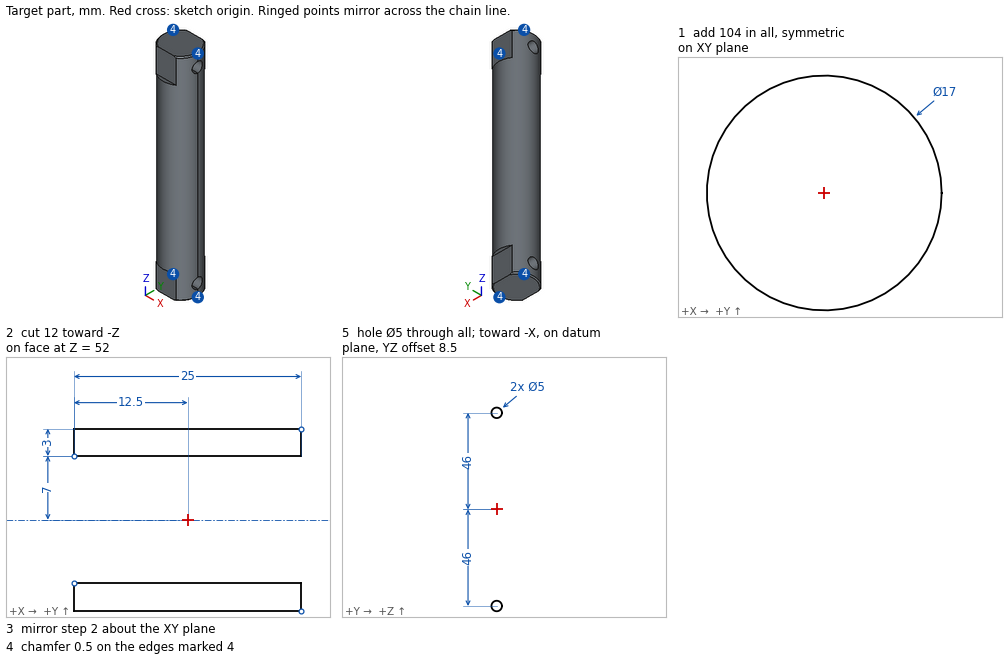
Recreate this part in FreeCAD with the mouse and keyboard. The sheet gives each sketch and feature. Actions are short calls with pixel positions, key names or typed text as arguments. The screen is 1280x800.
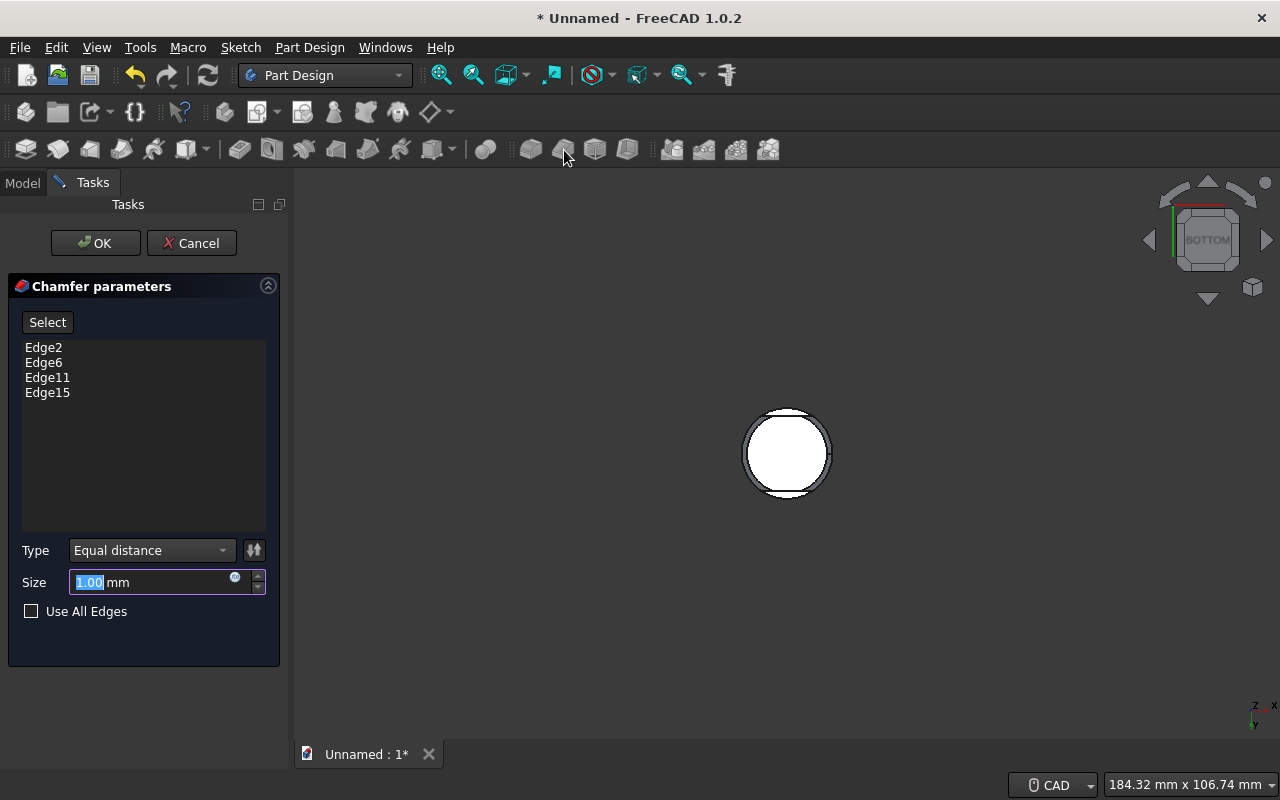
text(0.5)
key(Tab)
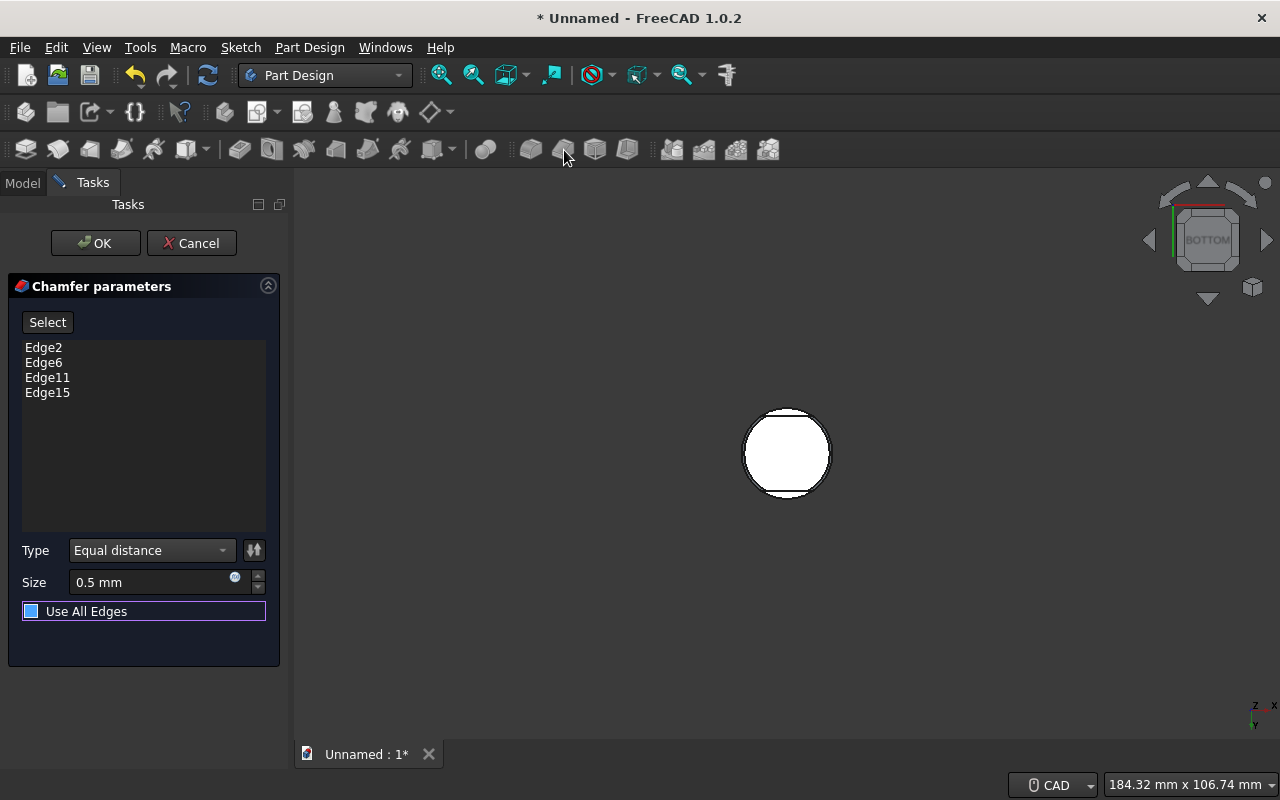
click(96, 243)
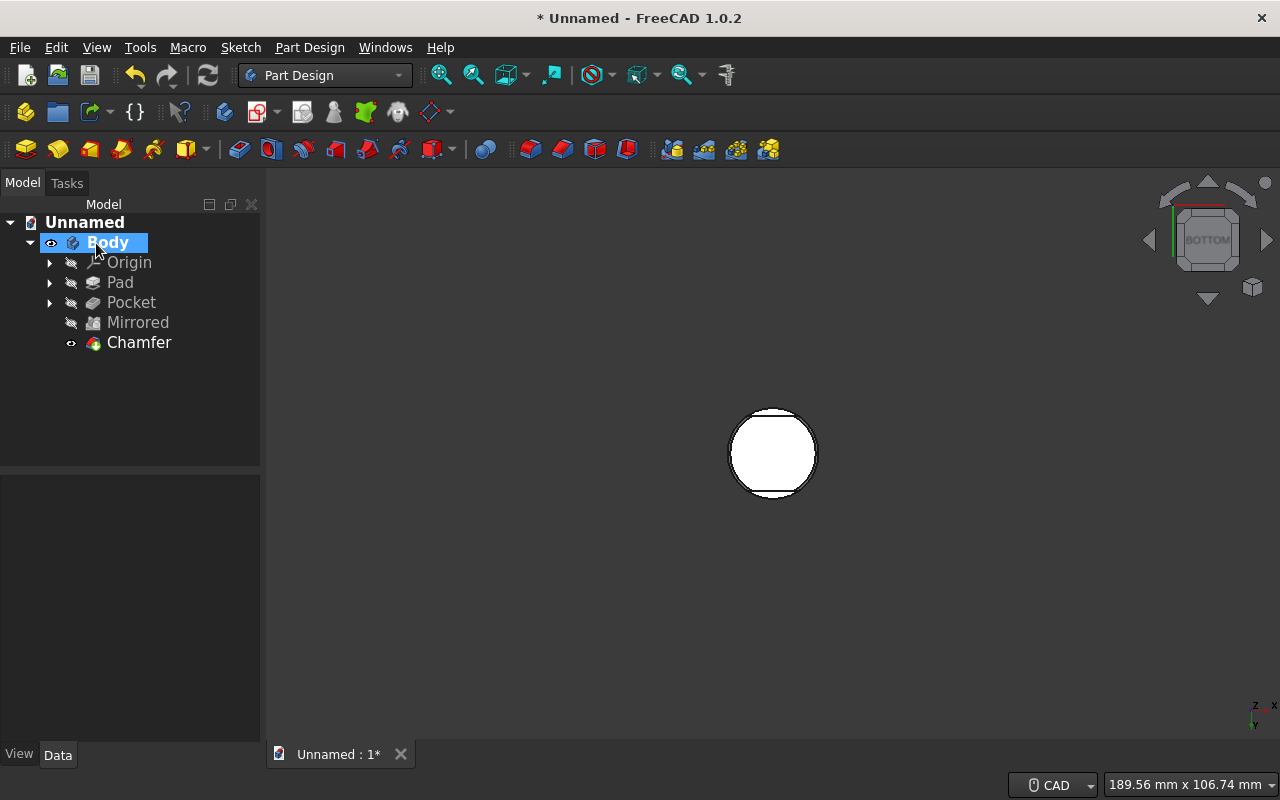
click(442, 76)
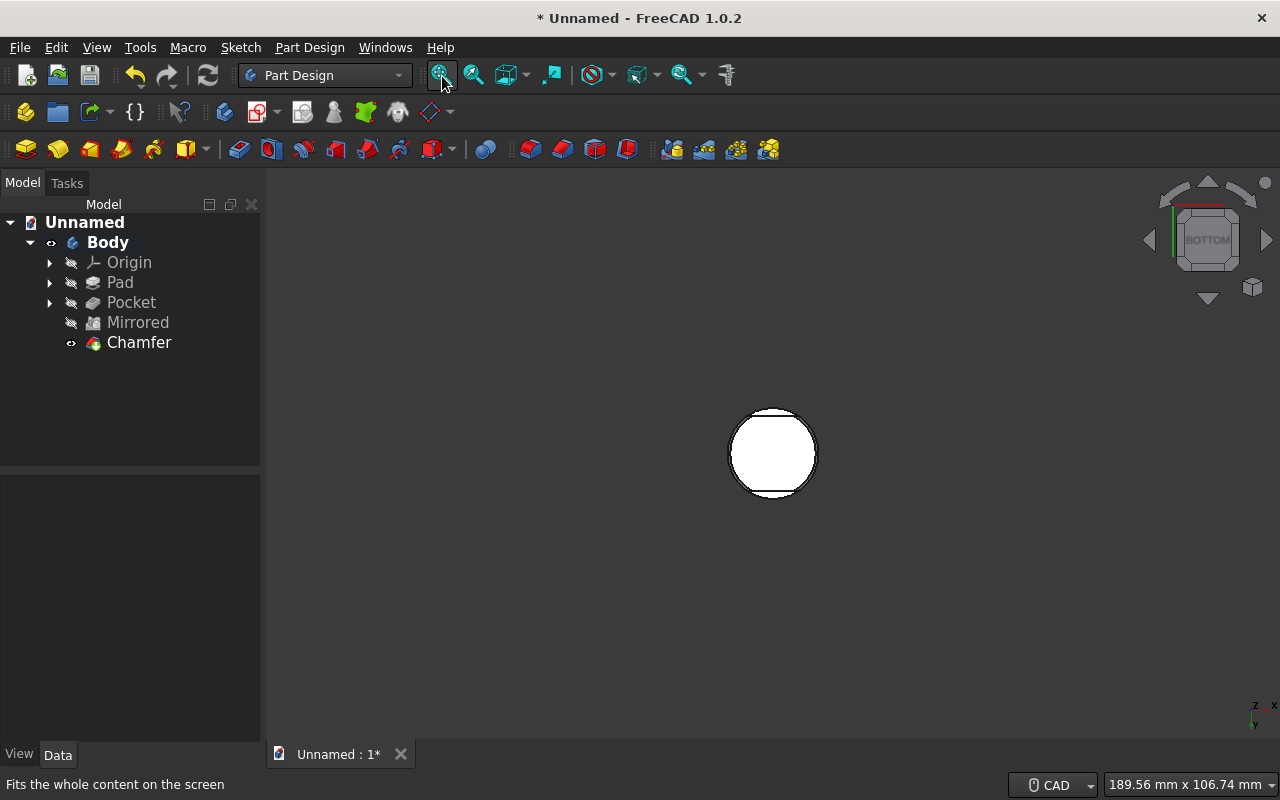
click(50, 263)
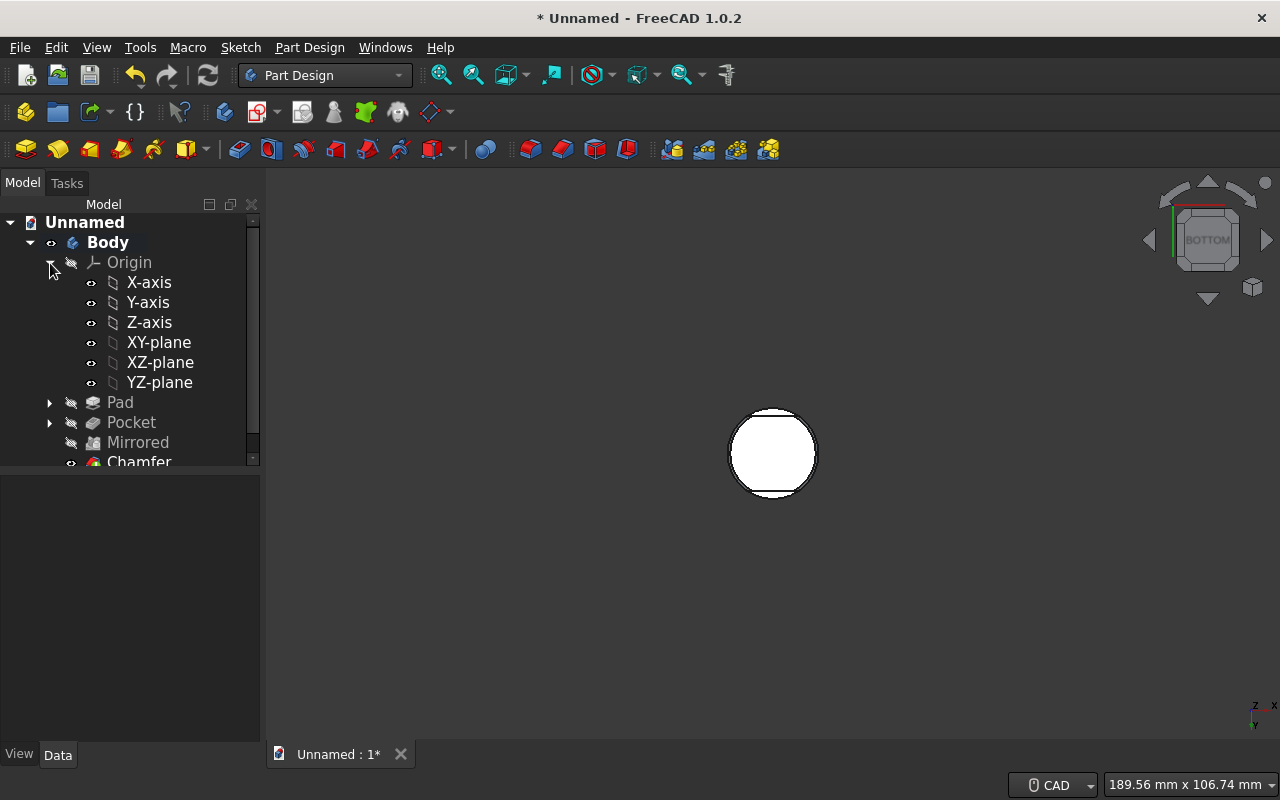
click(136, 383)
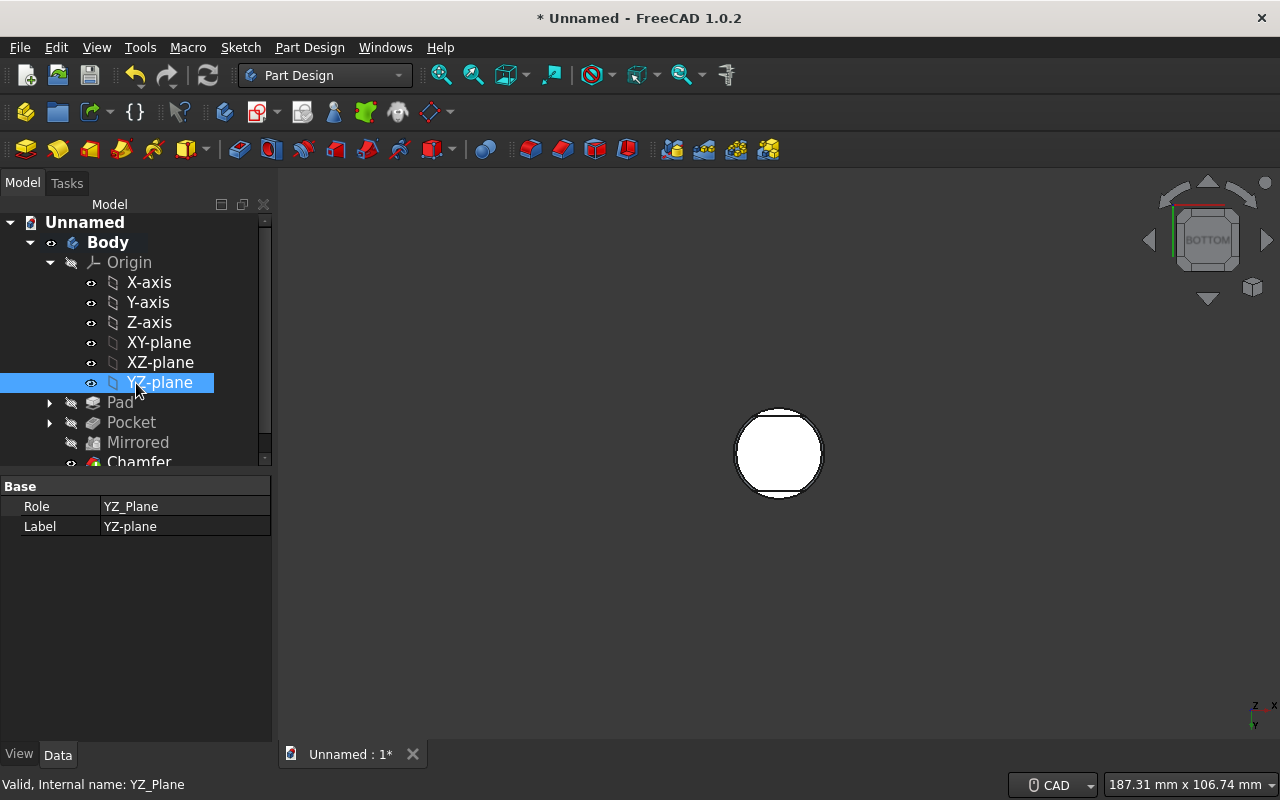
click(430, 112)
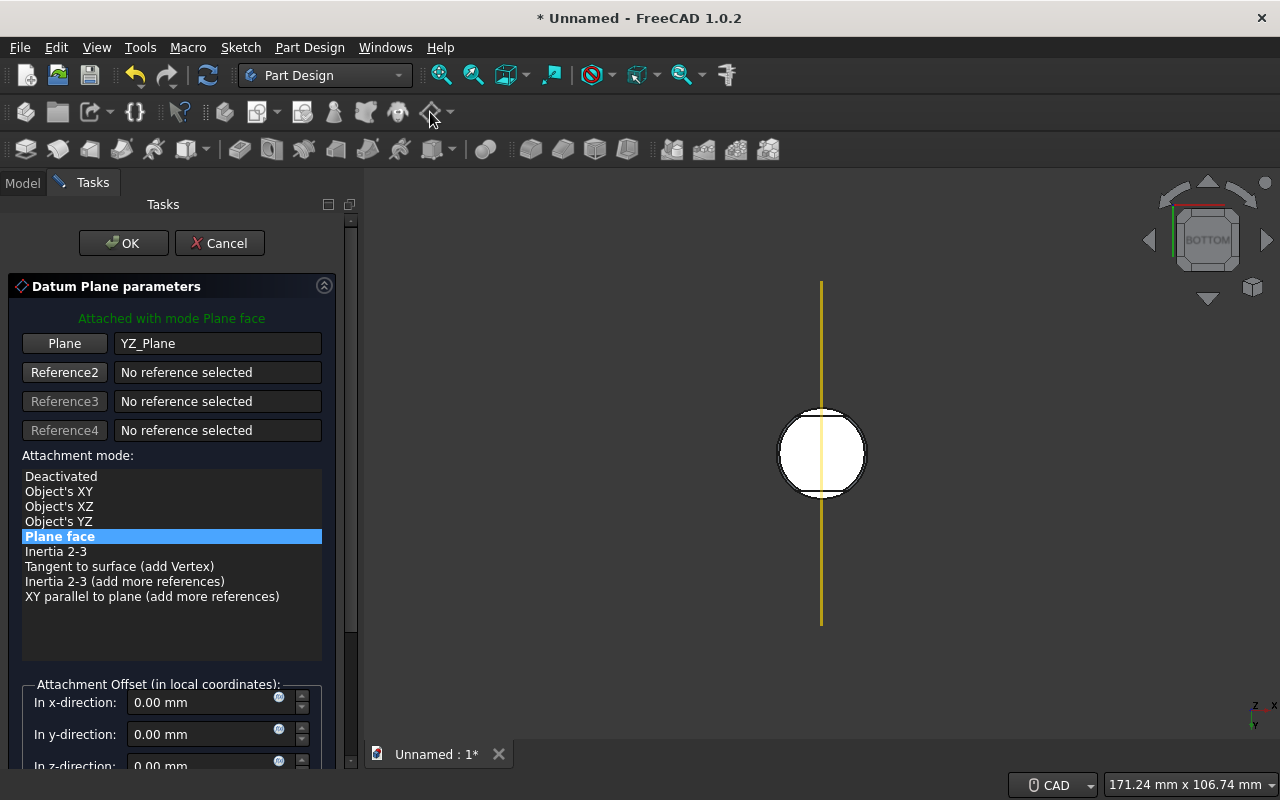
scroll(351, 491, down, 2)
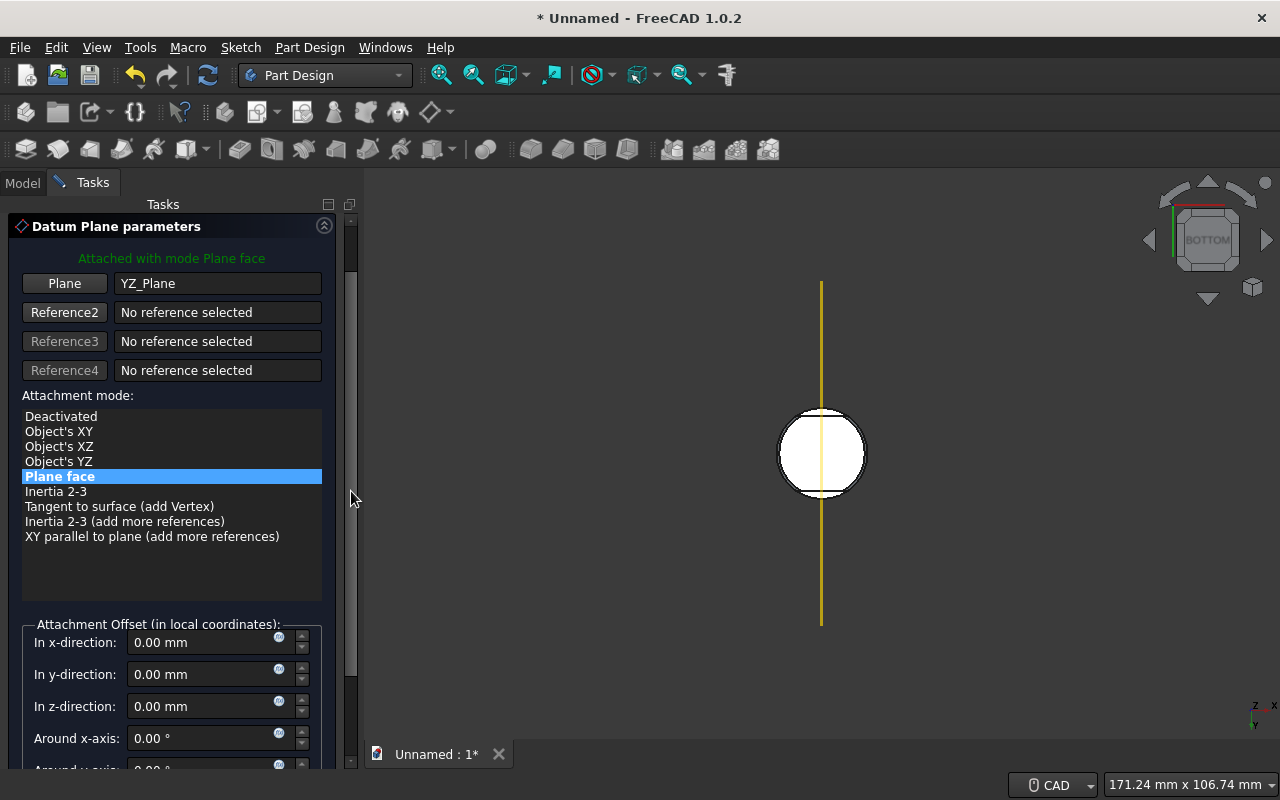
triple_click(210, 646)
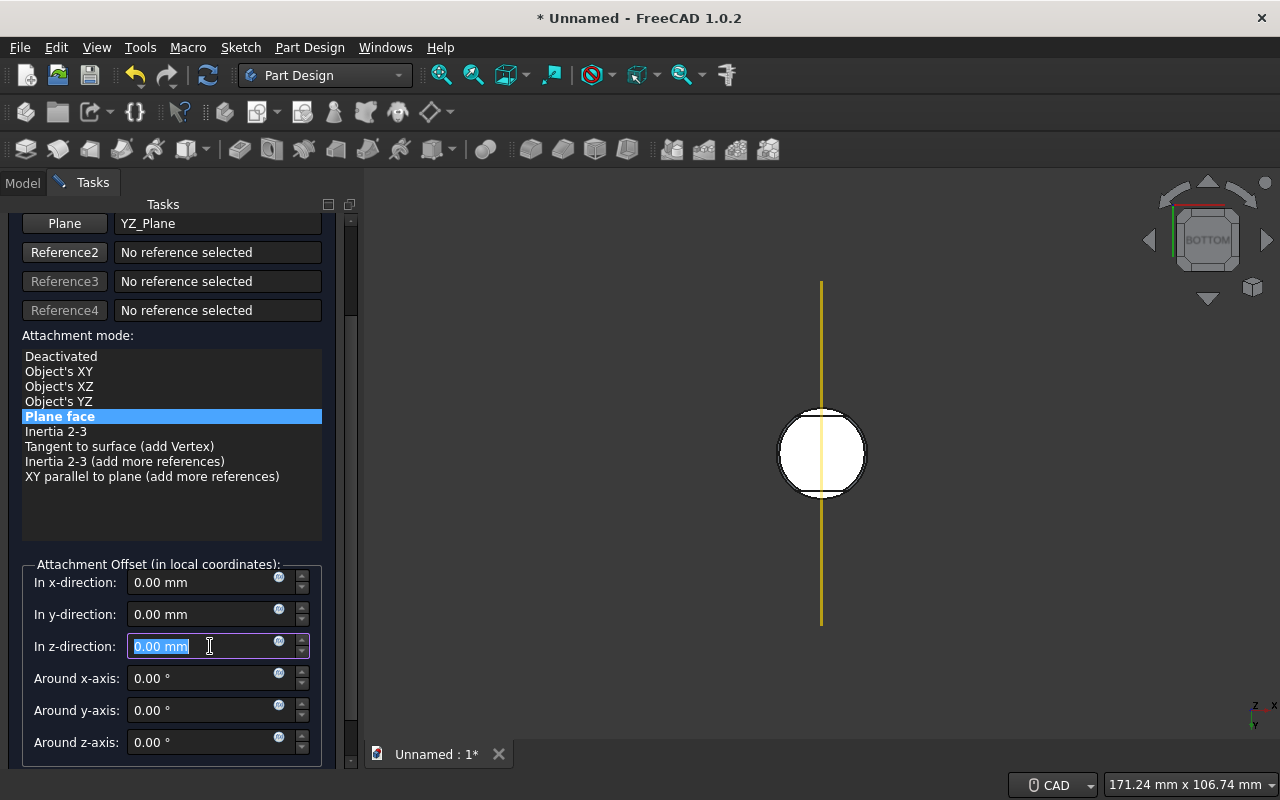
text(8.5)
key(Tab)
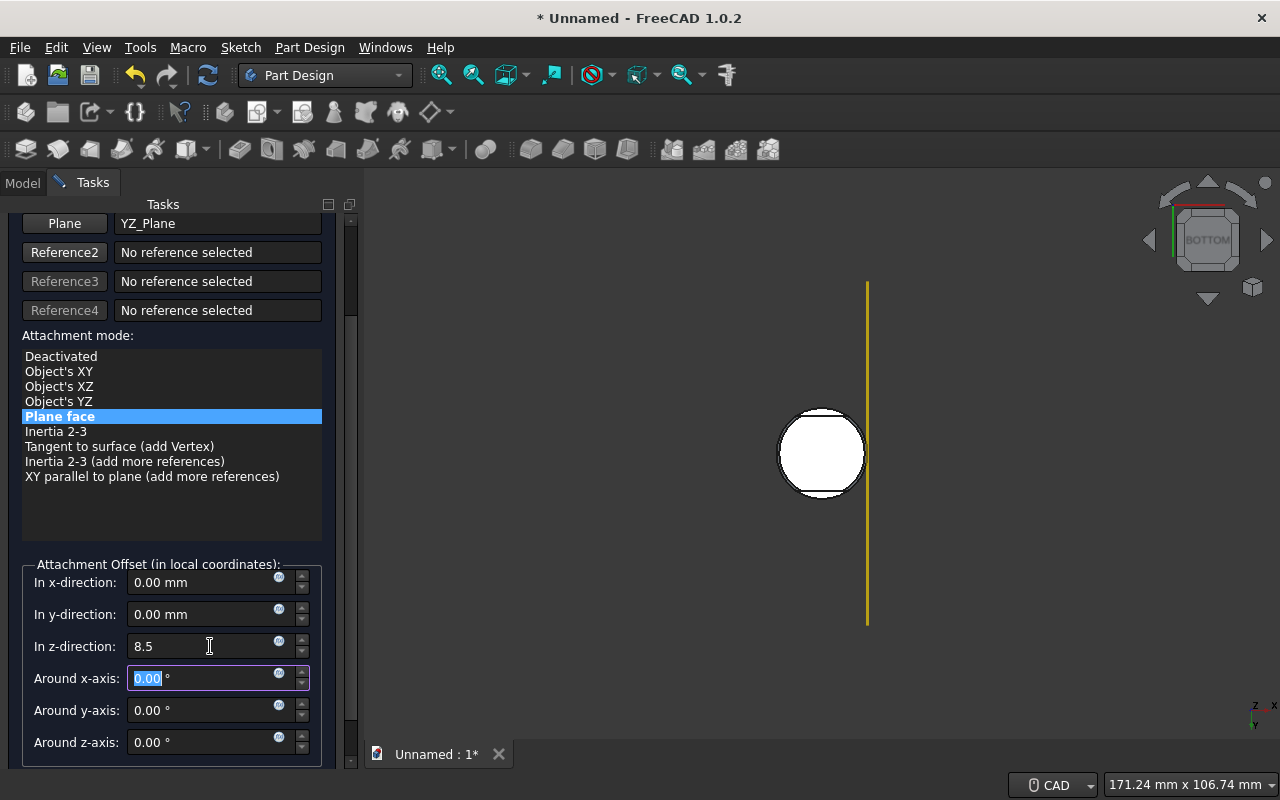
scroll(351, 491, up, 3)